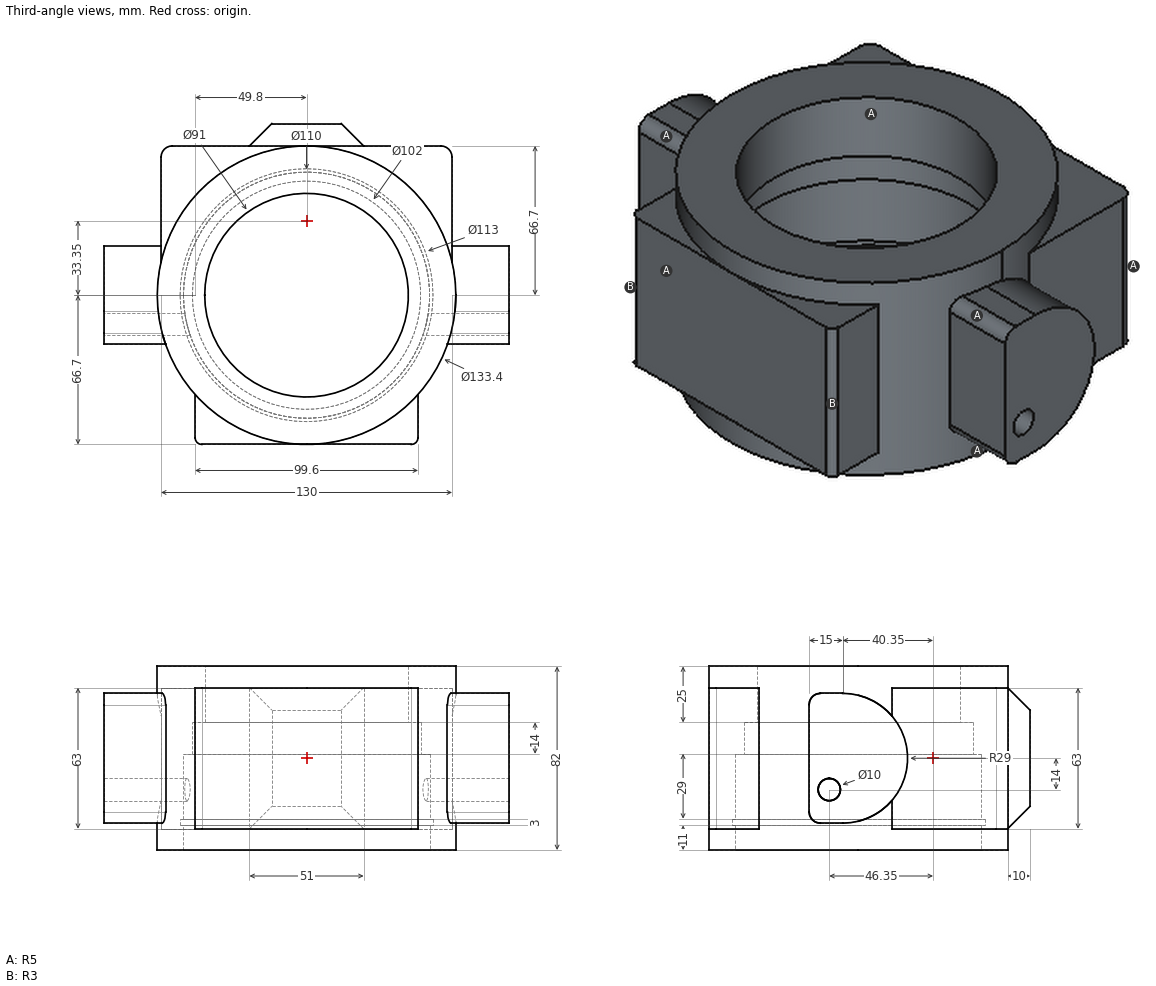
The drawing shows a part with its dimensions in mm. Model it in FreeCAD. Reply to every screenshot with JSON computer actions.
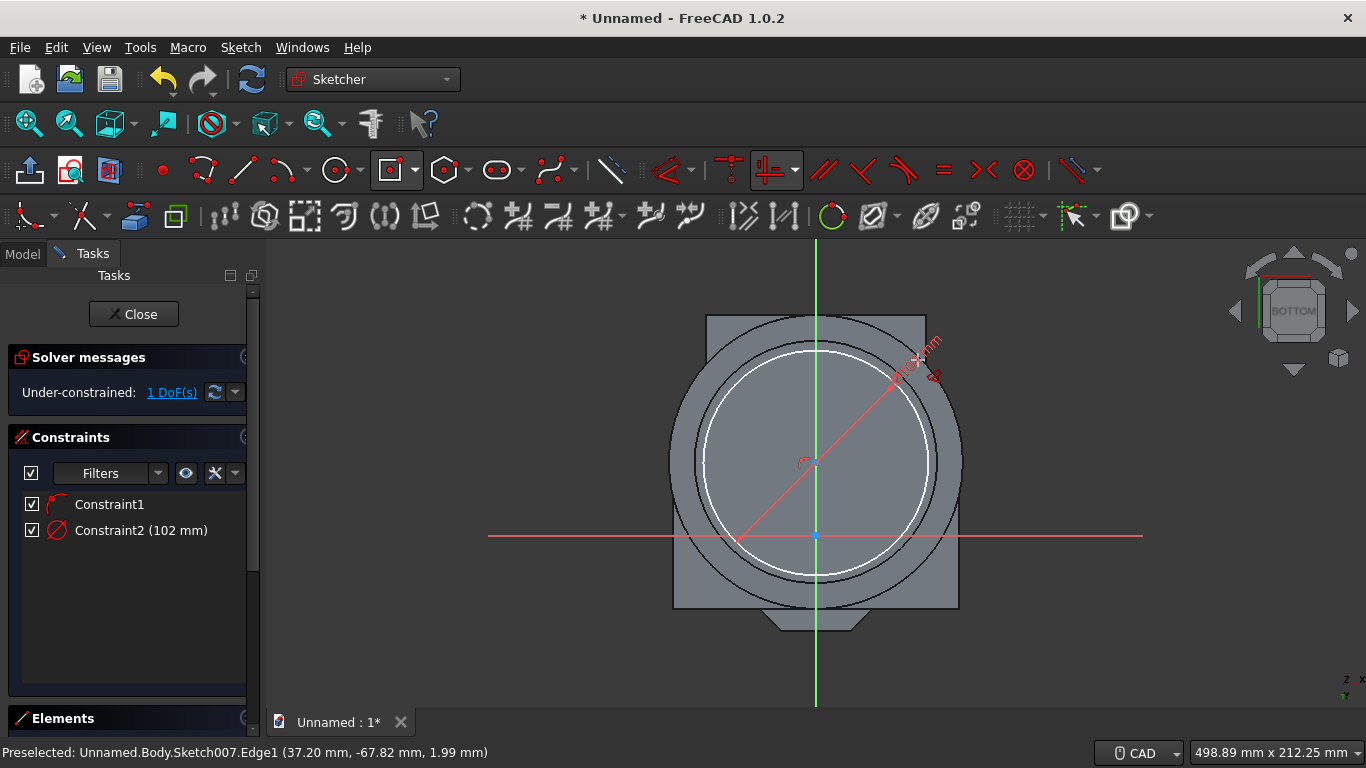
{"action": "left_click", "coordinate": [816, 463]}
{"action": "left_click", "coordinate": [850, 499]}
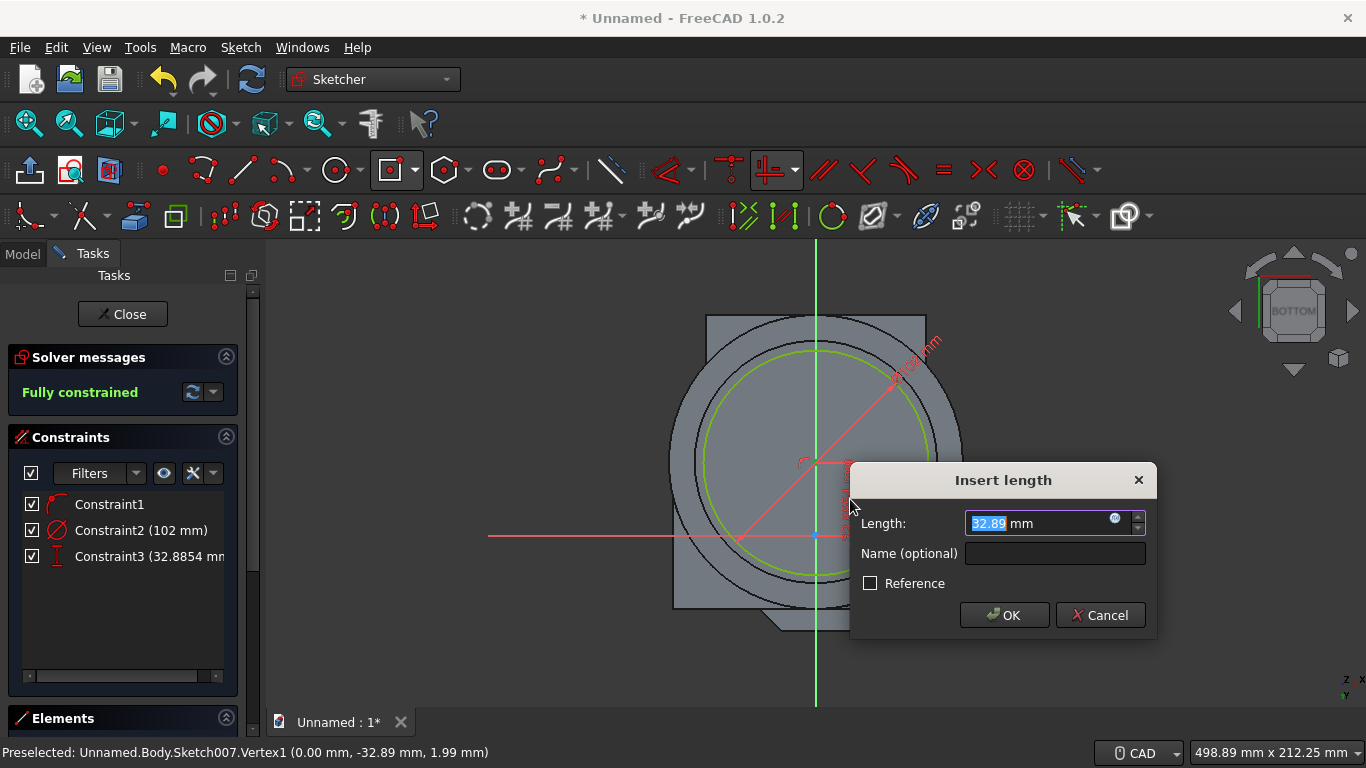
{"action": "type", "text": "33.35"}
{"action": "key", "text": "Return"}
{"action": "key", "text": "Escape"}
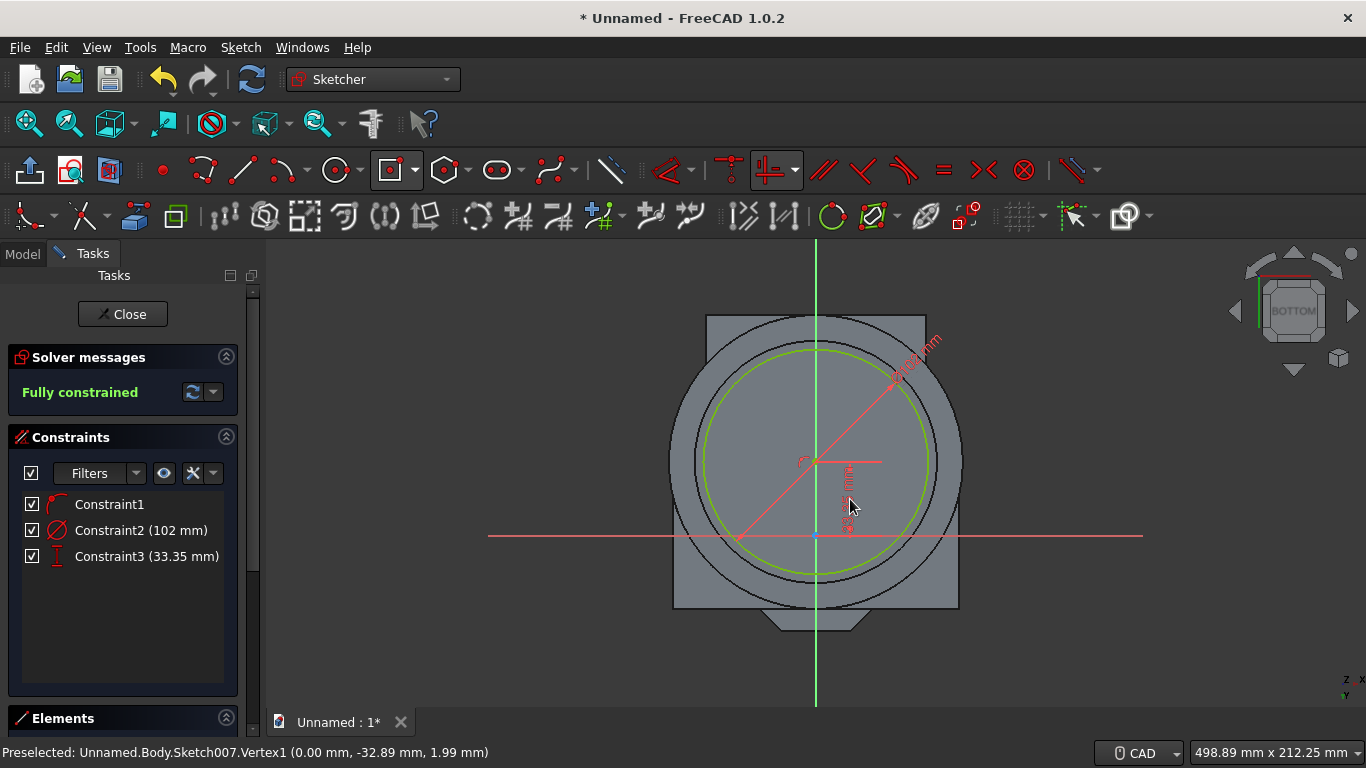
{"action": "left_click", "coordinate": [123, 314]}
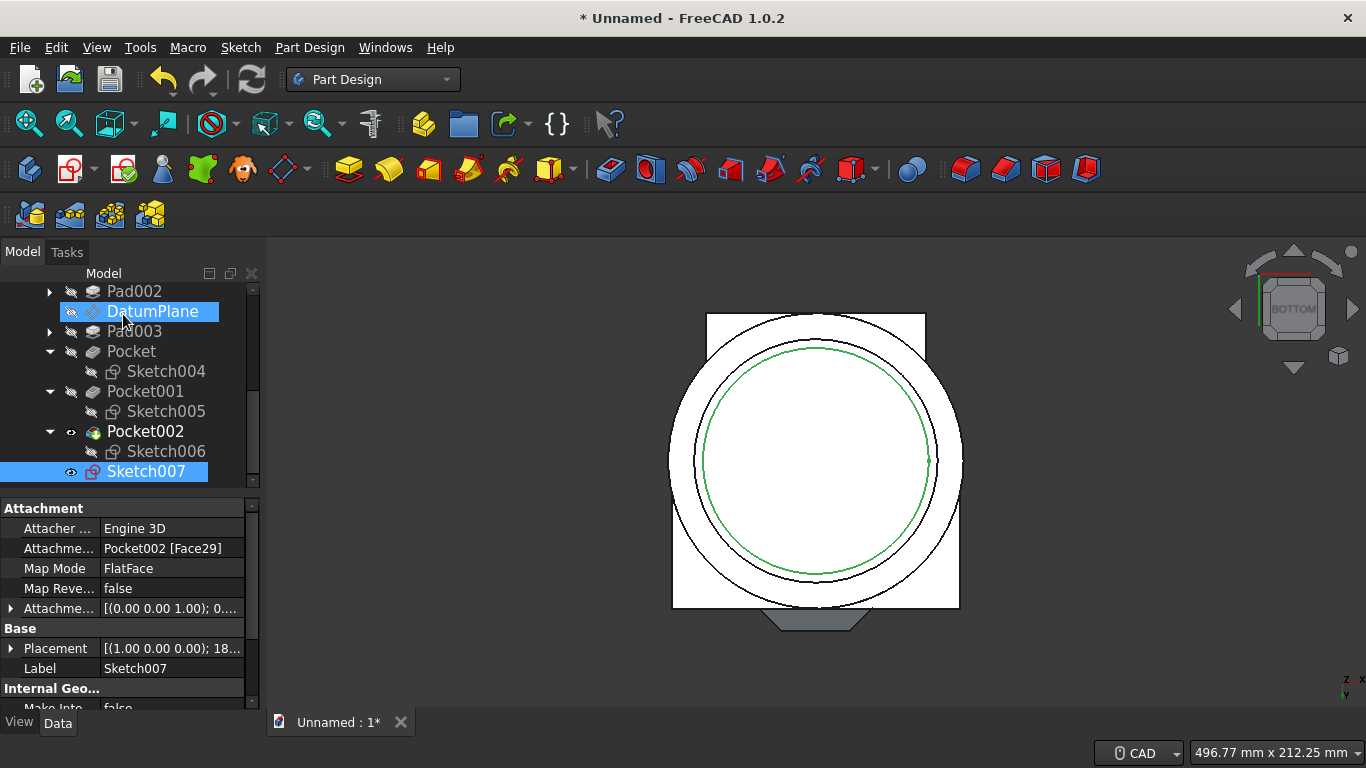
{"action": "left_click", "coordinate": [612, 170]}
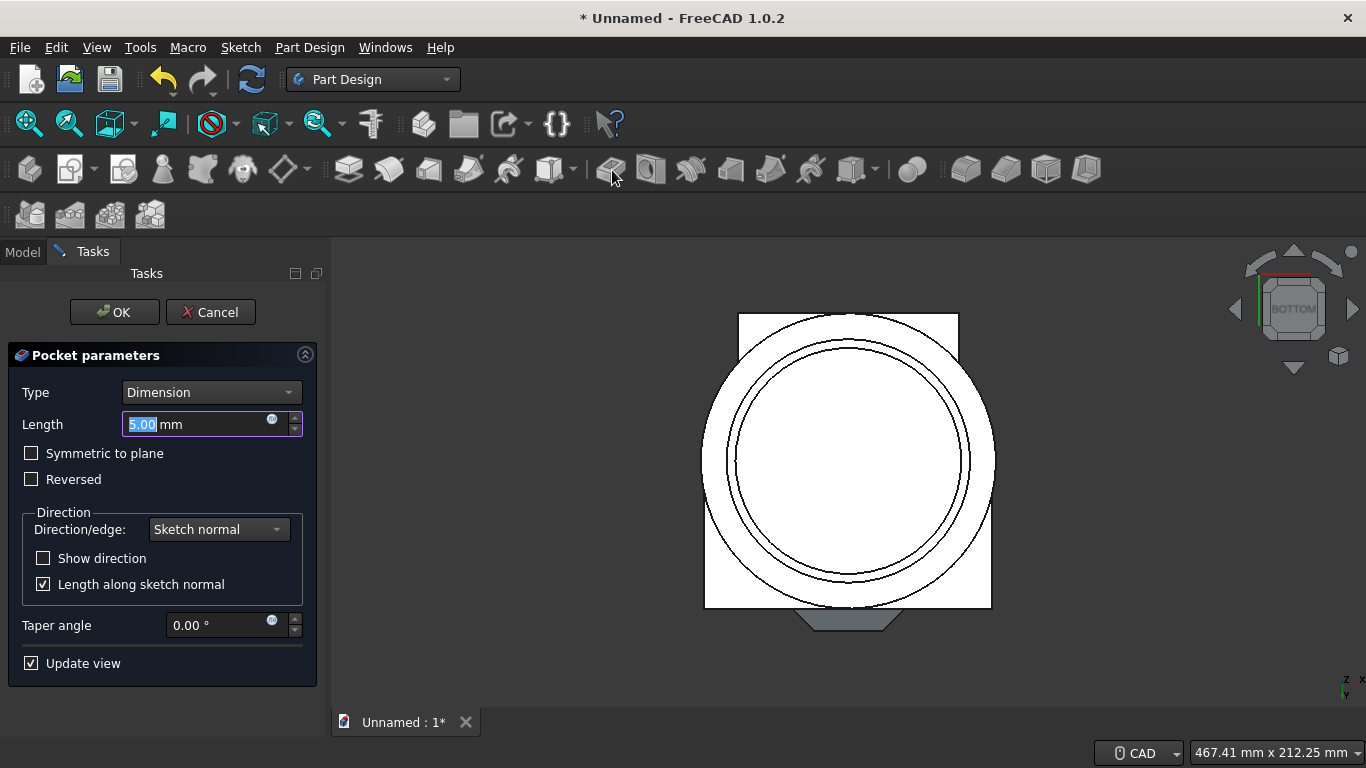
{"action": "type", "text": "14"}
{"action": "key", "text": "Tab"}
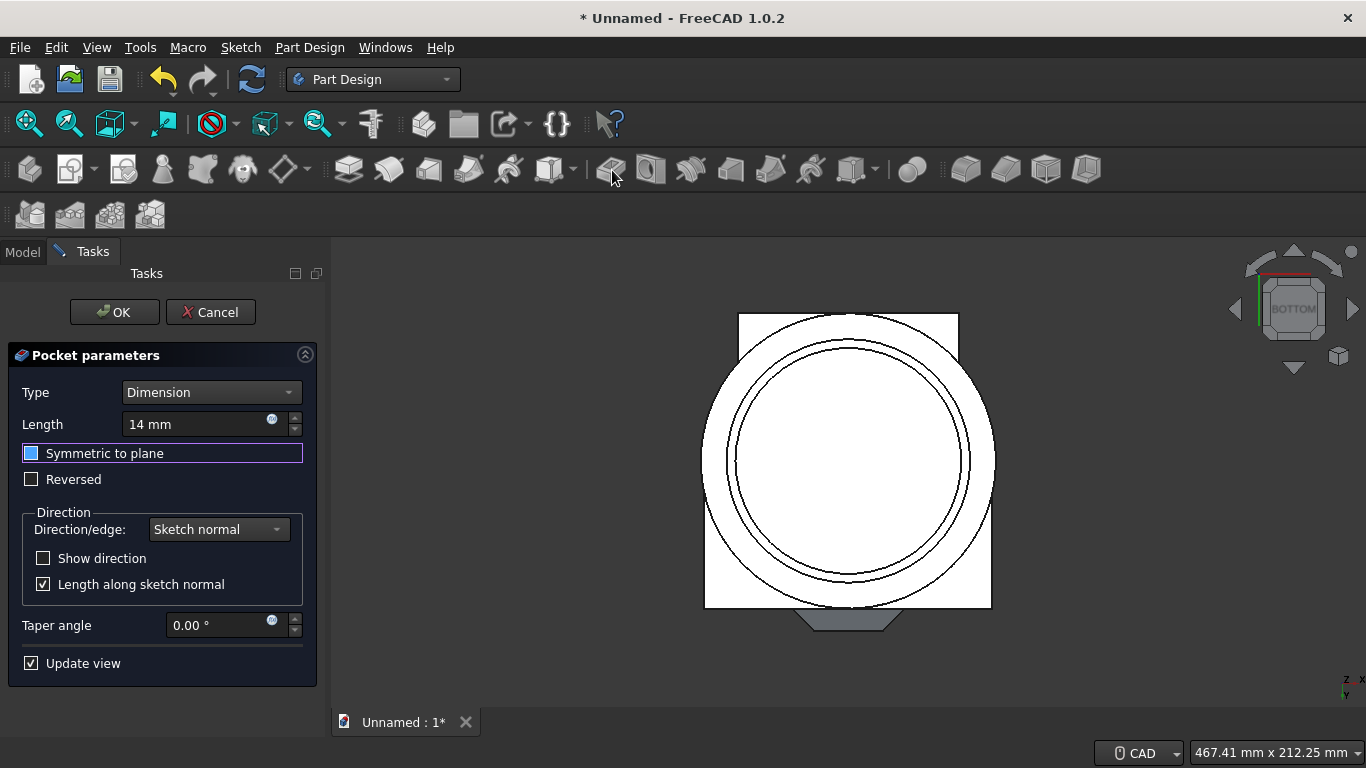
{"action": "left_click", "coordinate": [115, 312]}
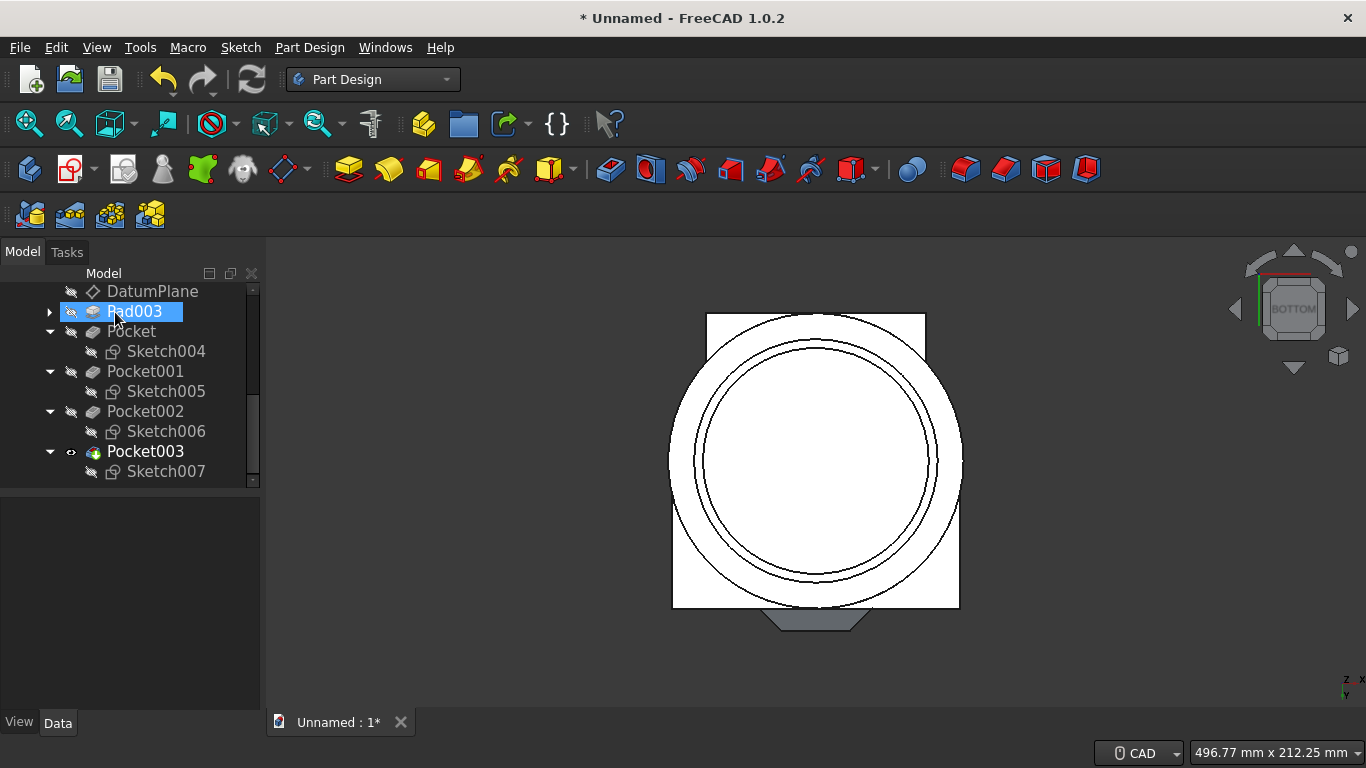
{"action": "left_click", "coordinate": [816, 460]}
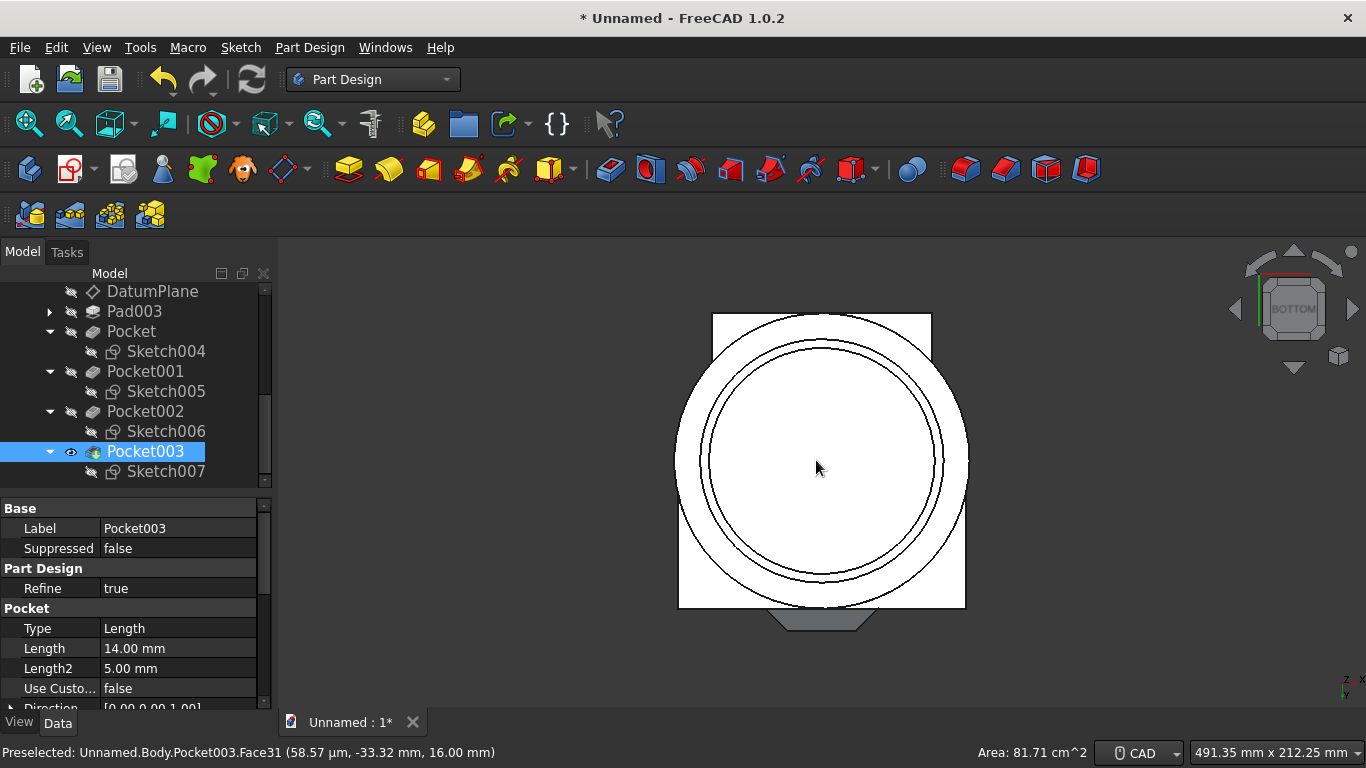
{"action": "left_click", "coordinate": [70, 170]}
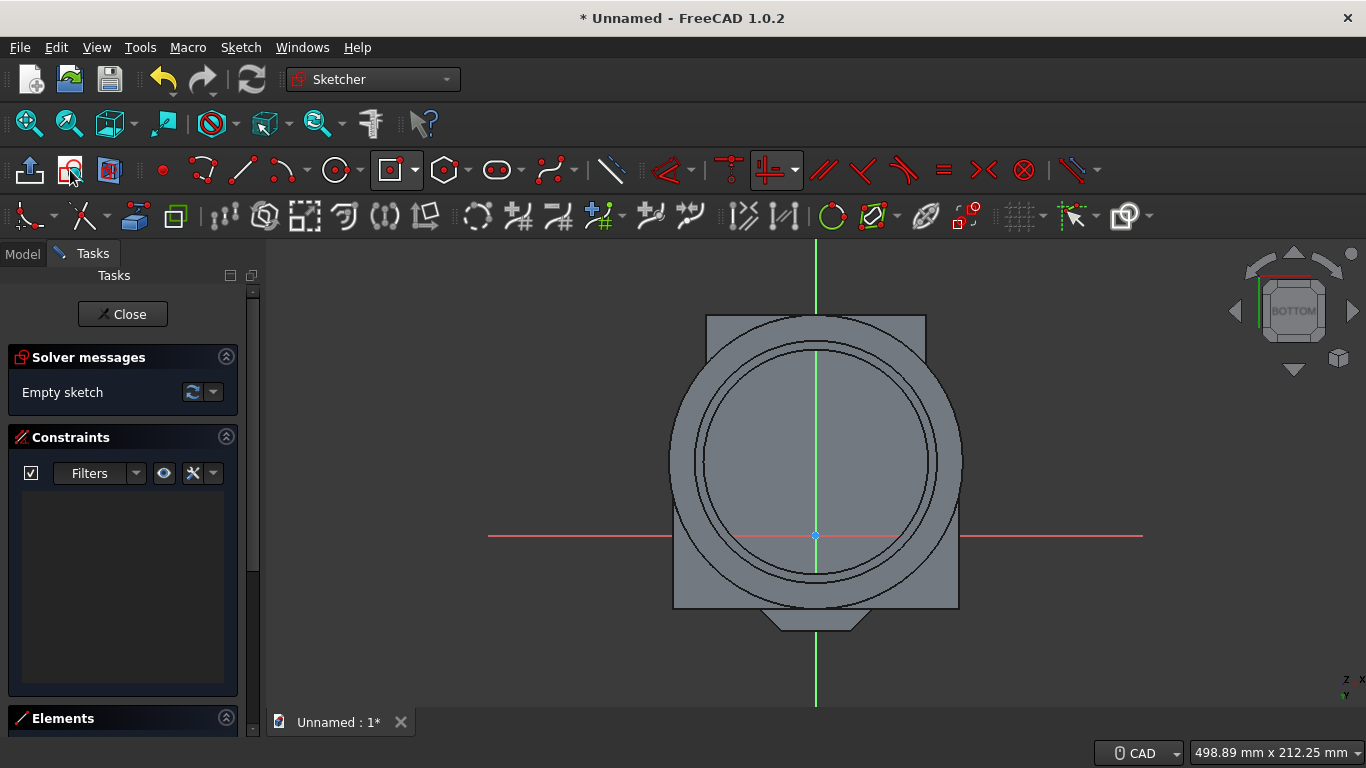
{"action": "key", "text": "q s"}